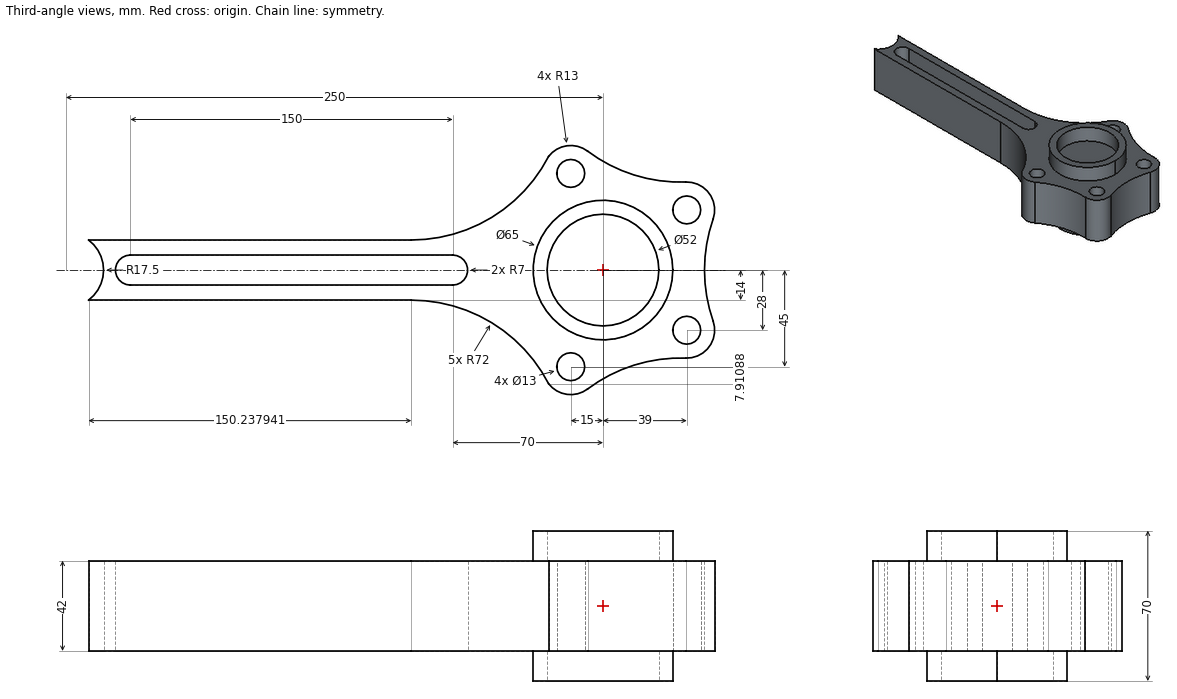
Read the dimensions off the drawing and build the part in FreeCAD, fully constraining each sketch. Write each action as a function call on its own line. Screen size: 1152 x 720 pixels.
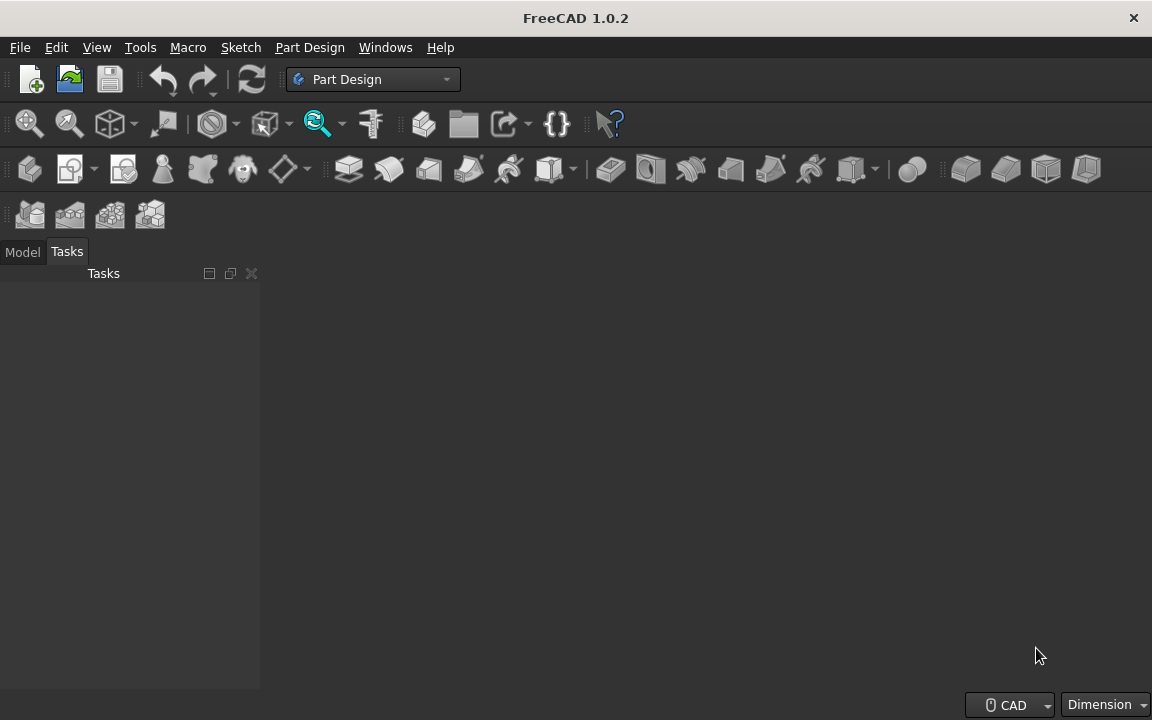
click(30, 80)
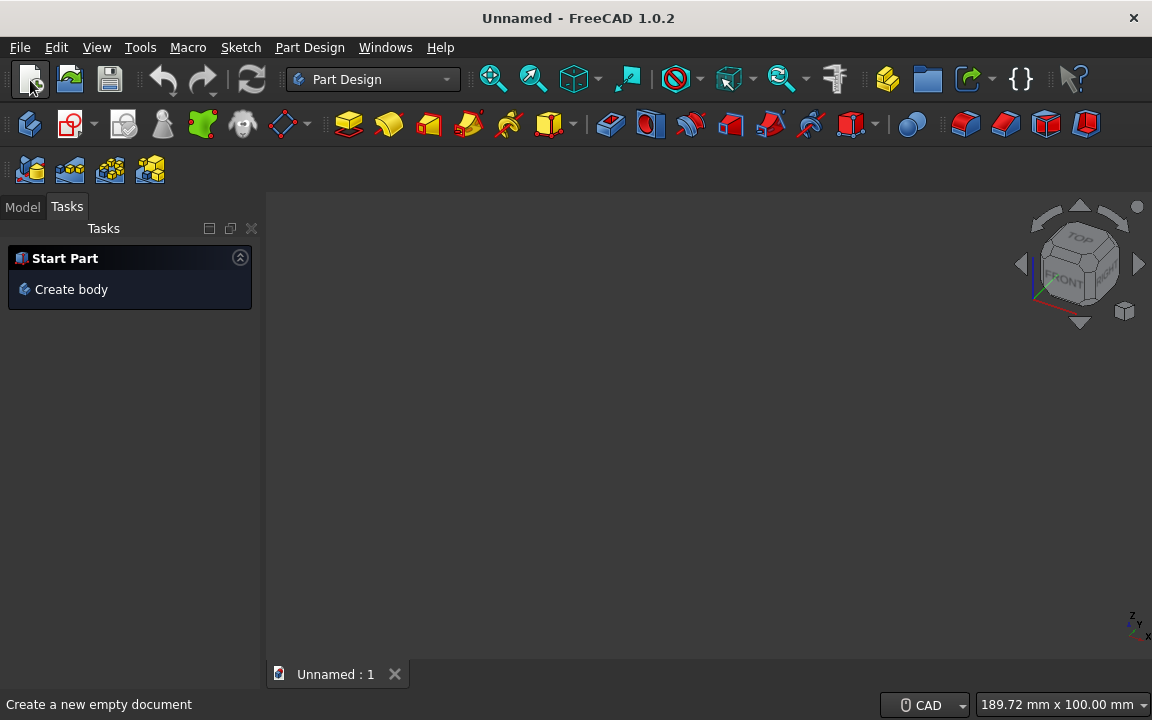
click(70, 124)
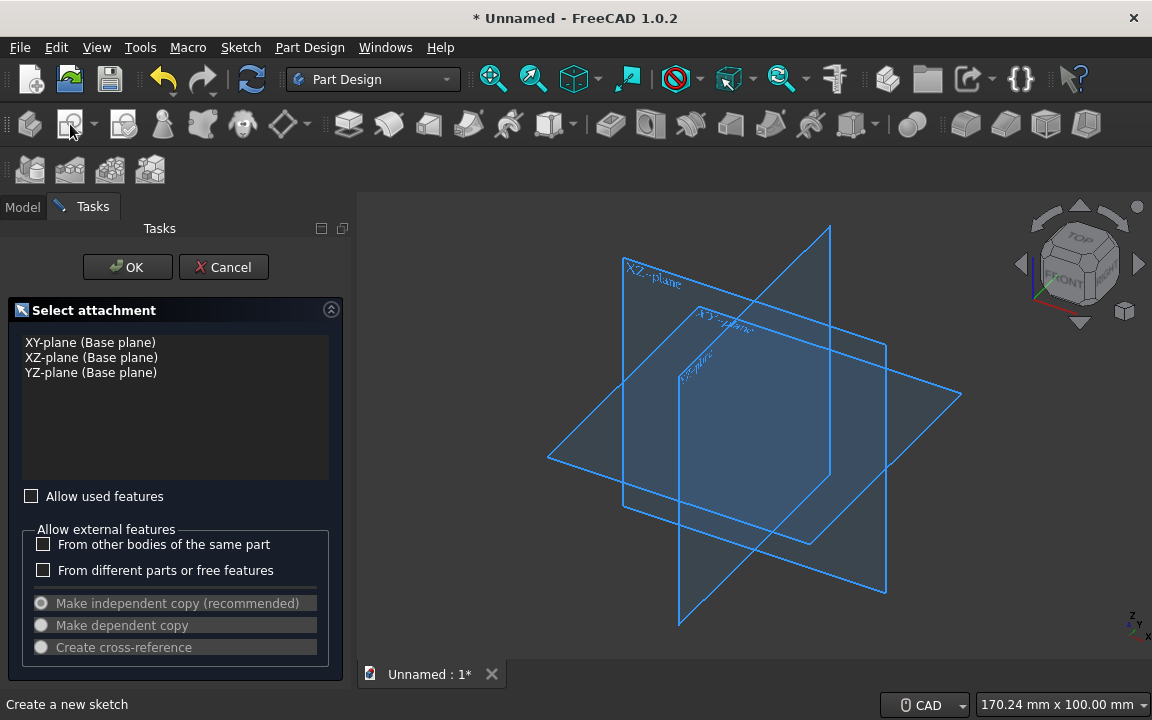
click(82, 342)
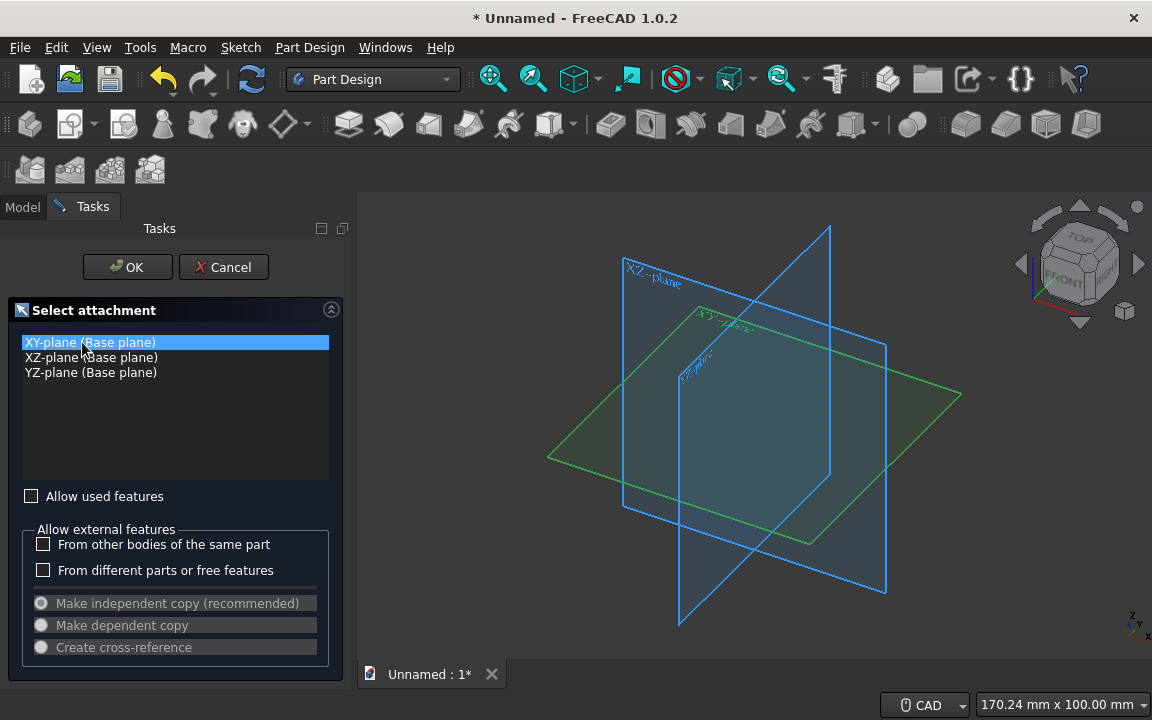
click(128, 267)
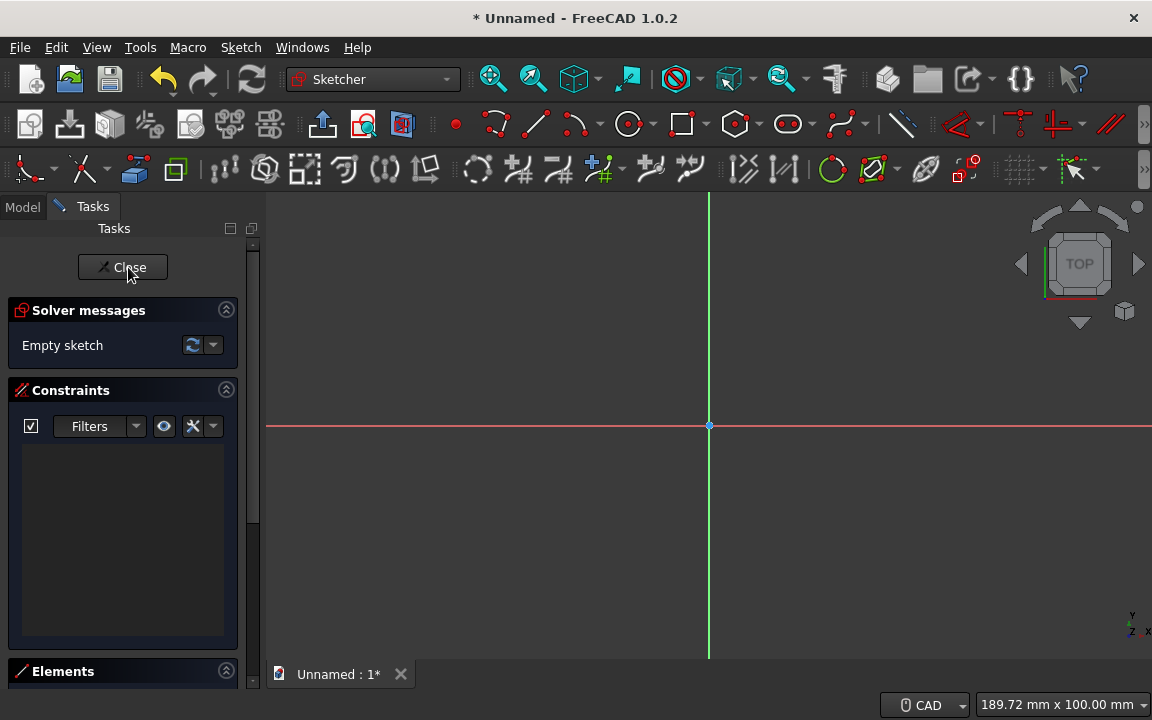
click(630, 124)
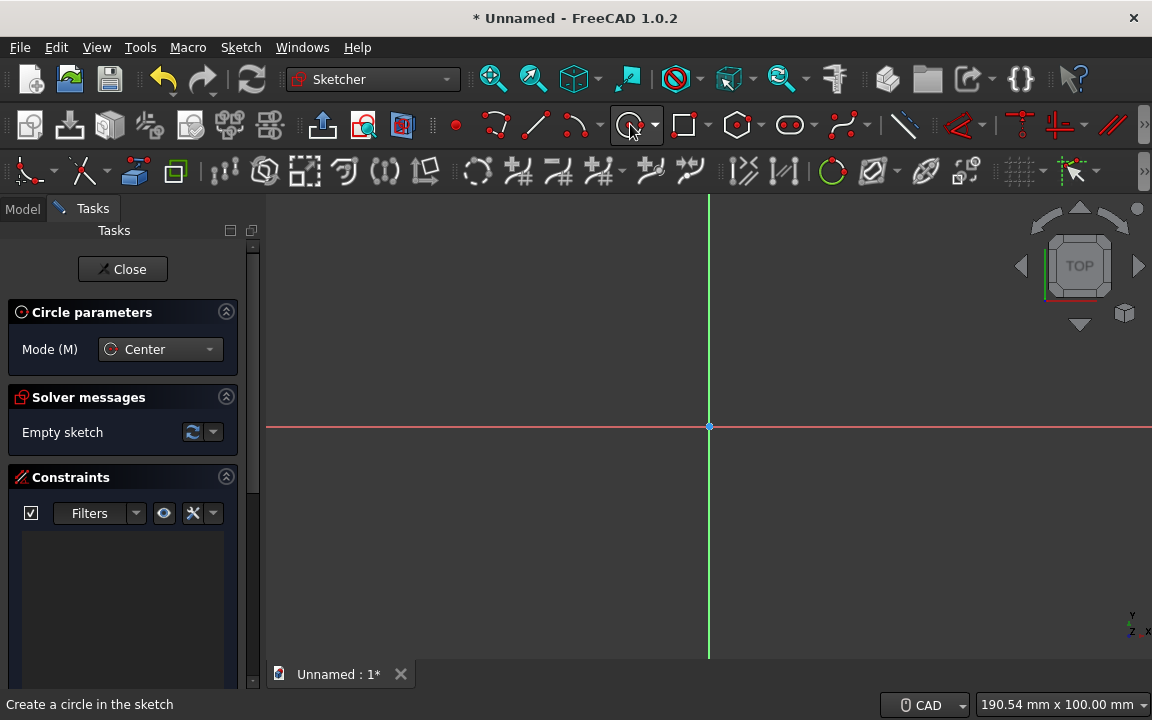
click(709, 426)
move(816, 320)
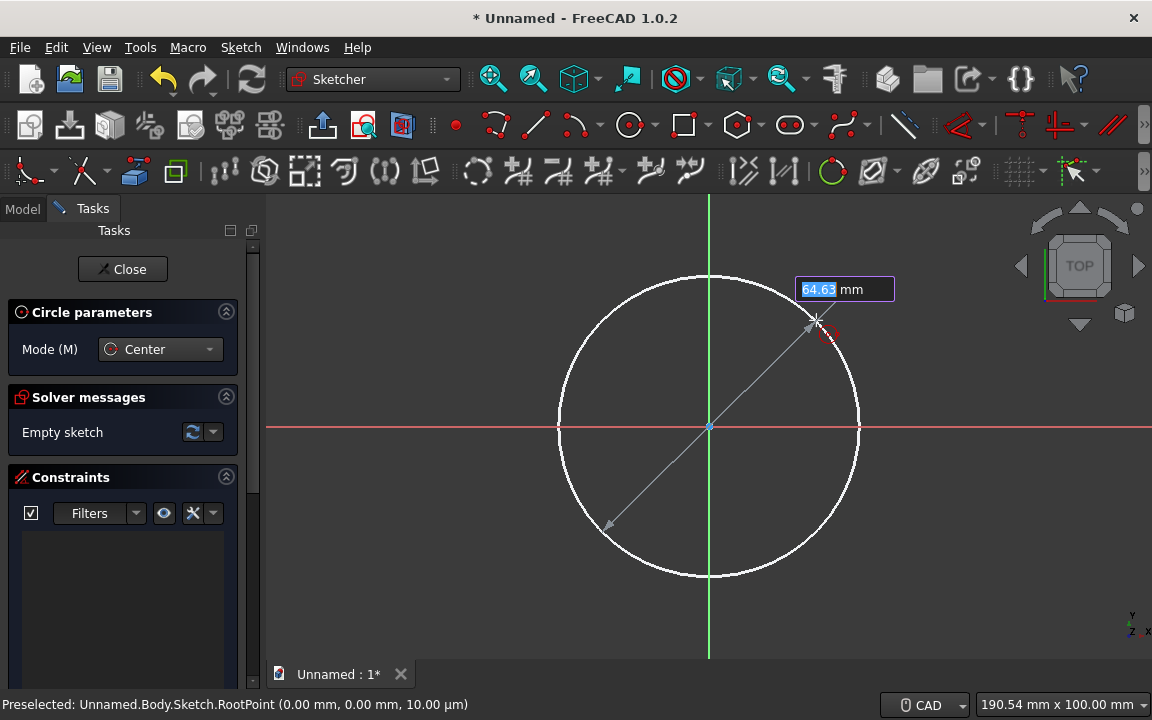
text(65)
key(Return)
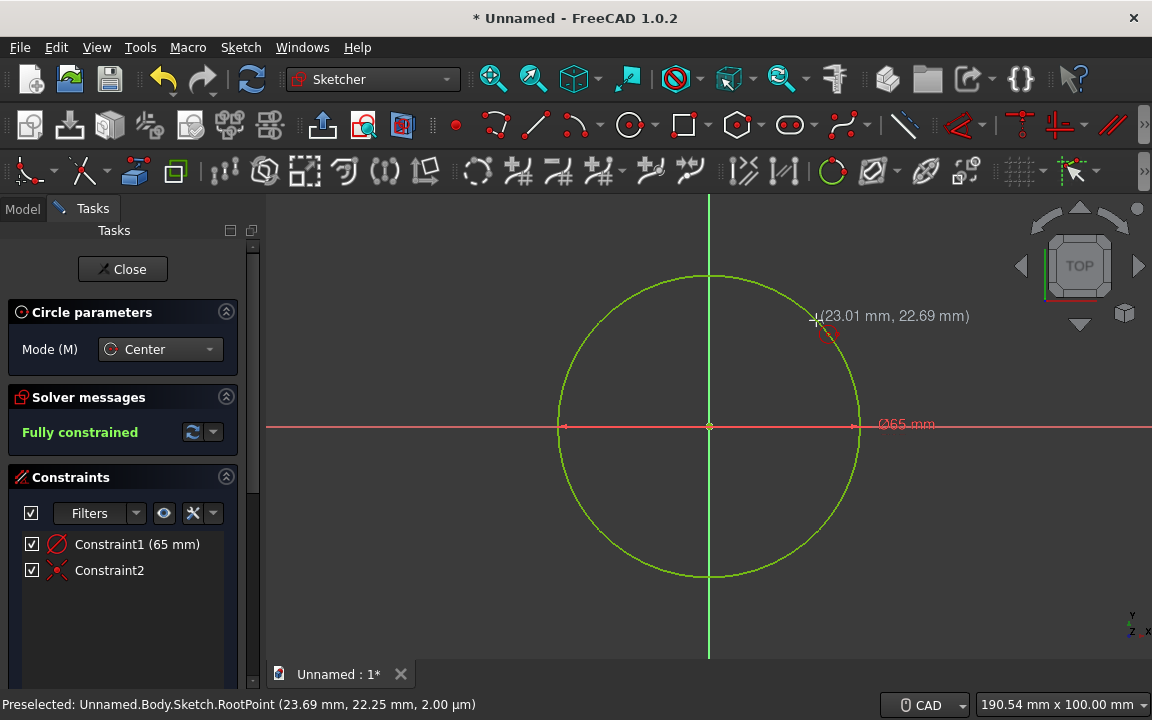
click(709, 426)
move(794, 341)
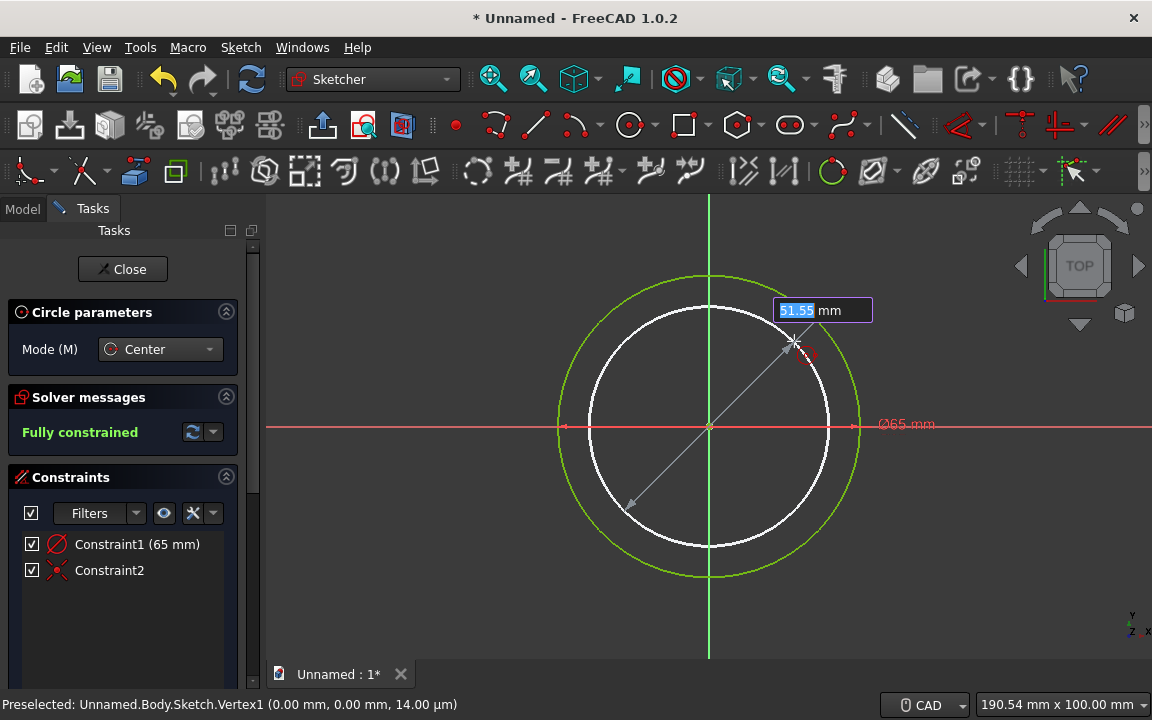
text(52)
key(Return)
key(Escape)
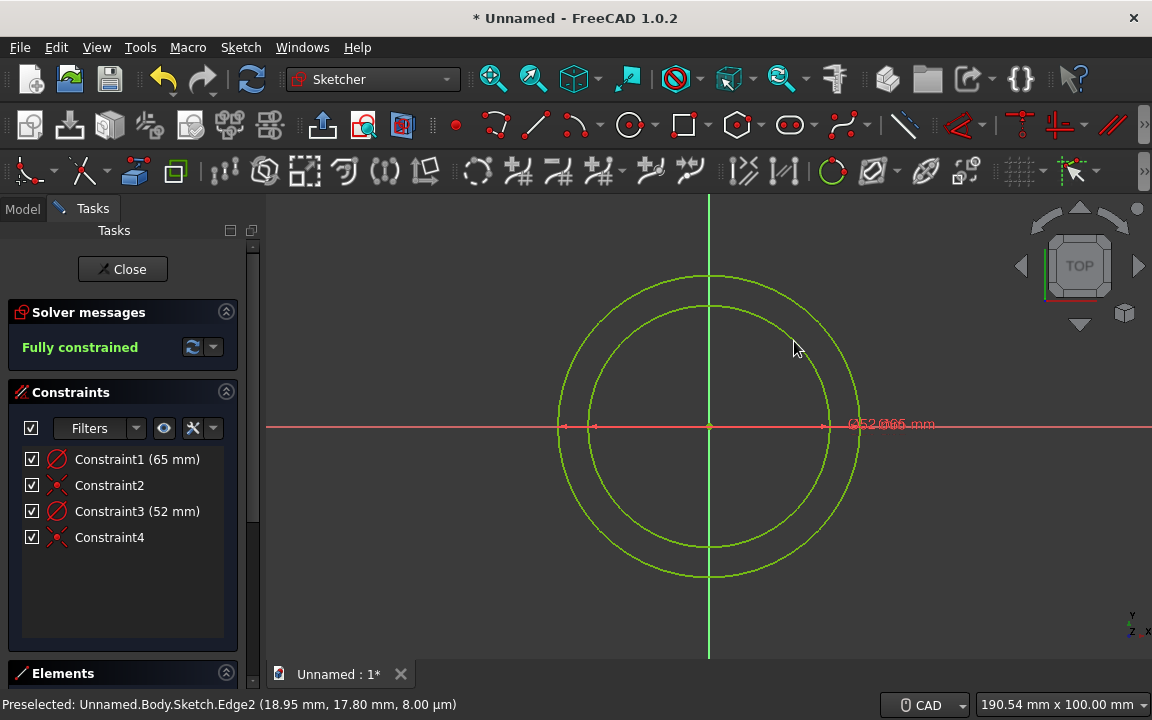
click(123, 269)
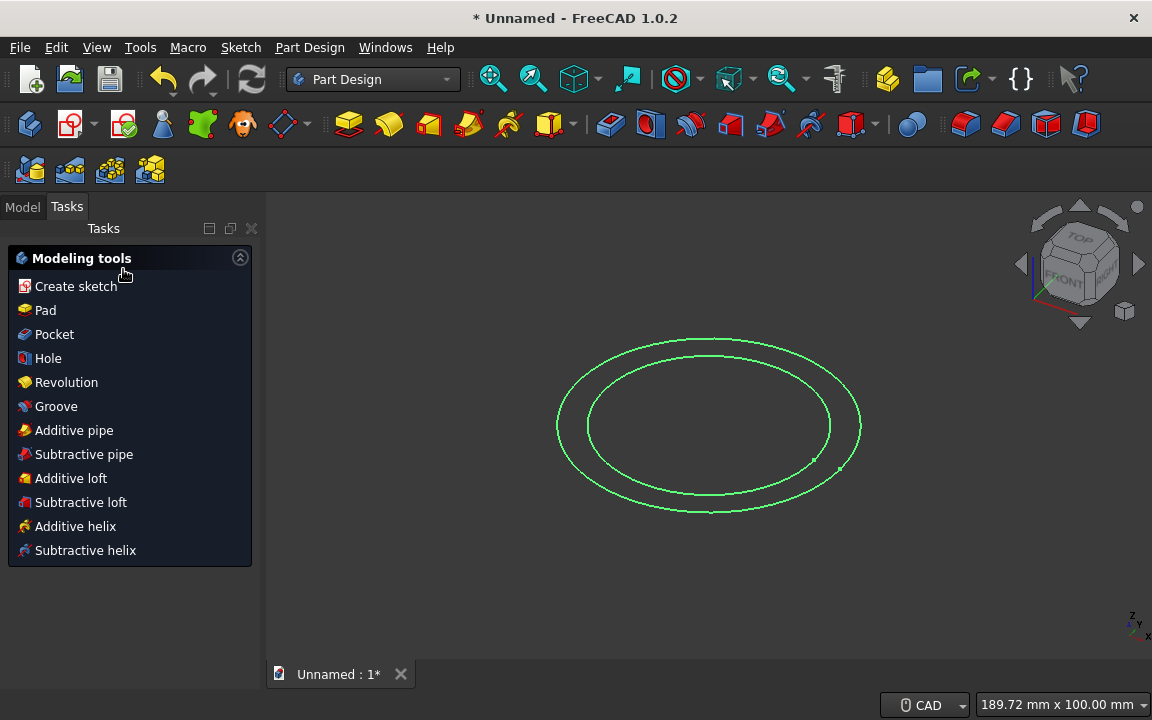
click(350, 124)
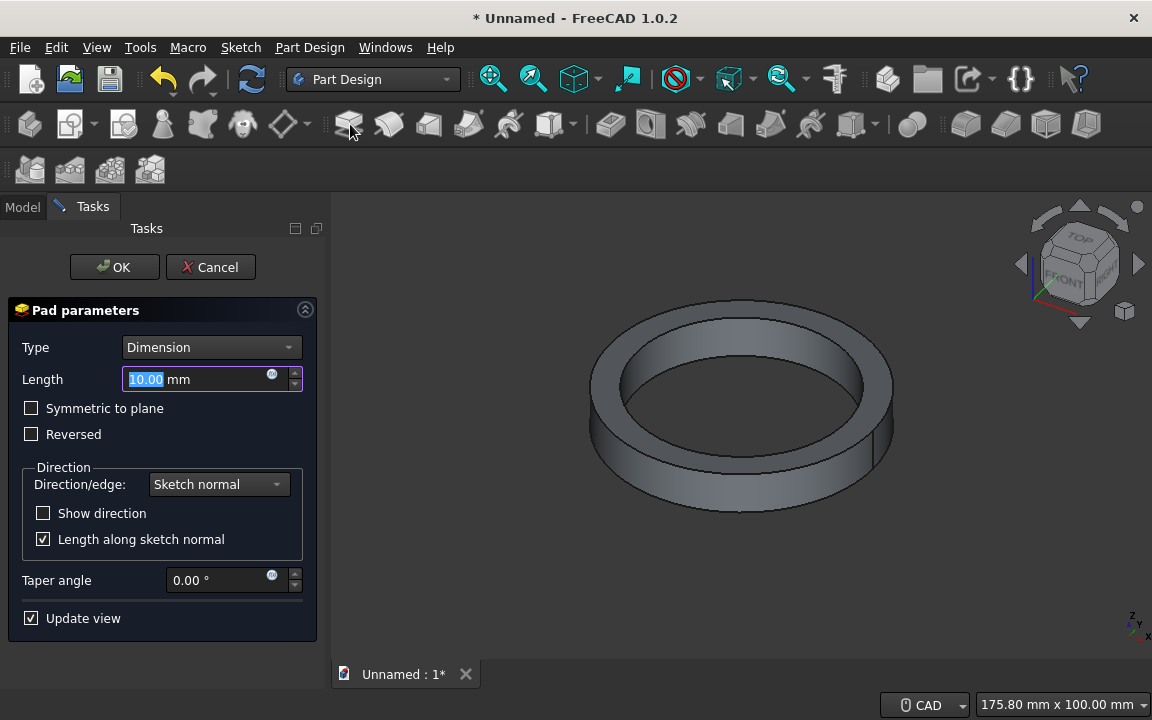
text(70)
key(Tab)